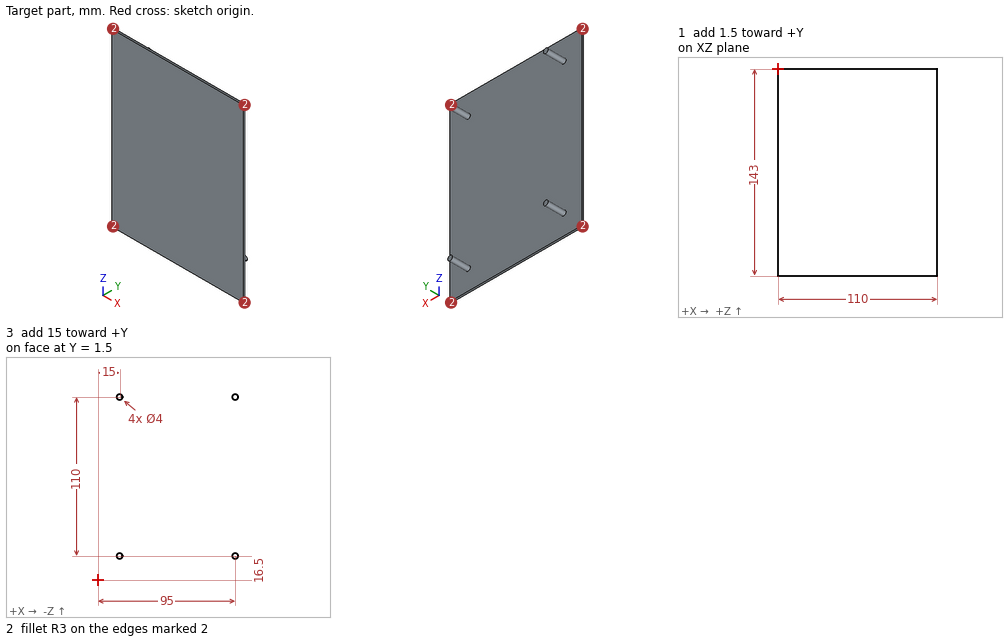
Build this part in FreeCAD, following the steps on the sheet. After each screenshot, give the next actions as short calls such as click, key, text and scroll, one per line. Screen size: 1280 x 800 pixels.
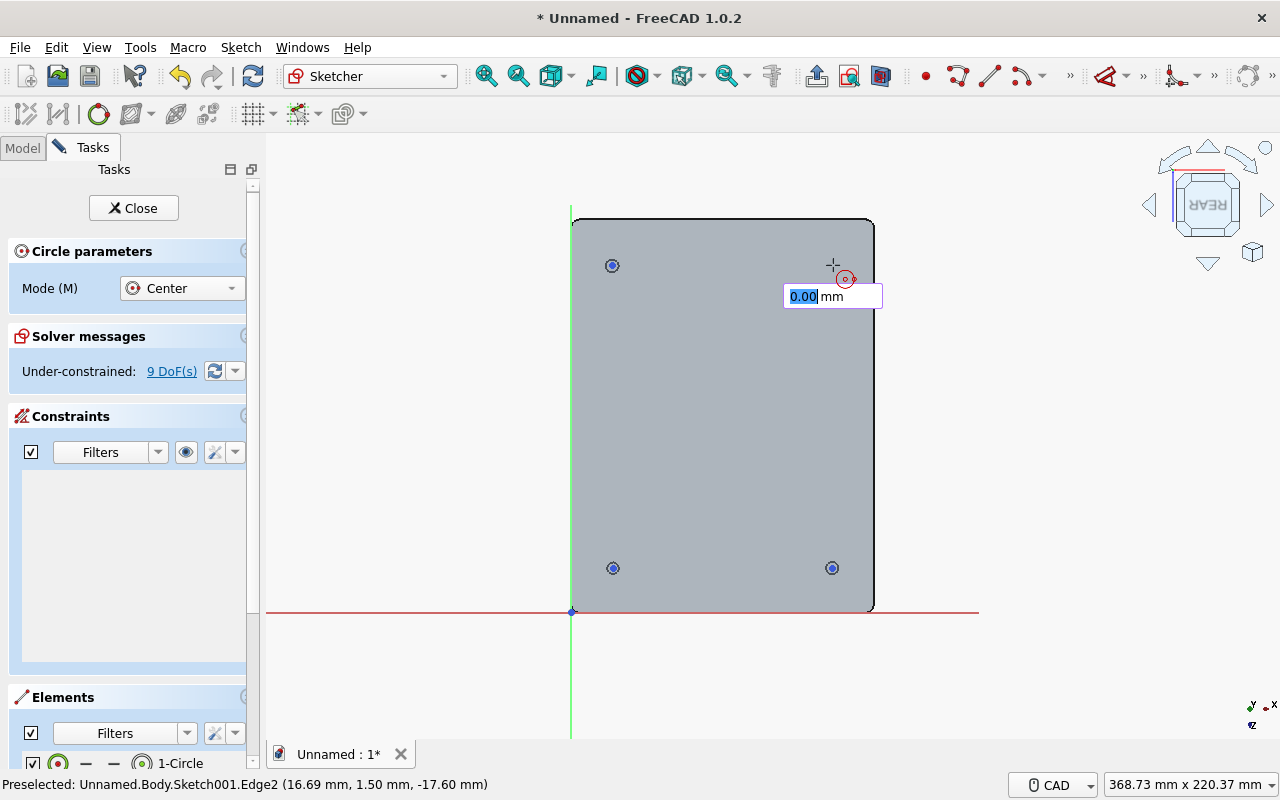
scroll(836, 261, up, 6)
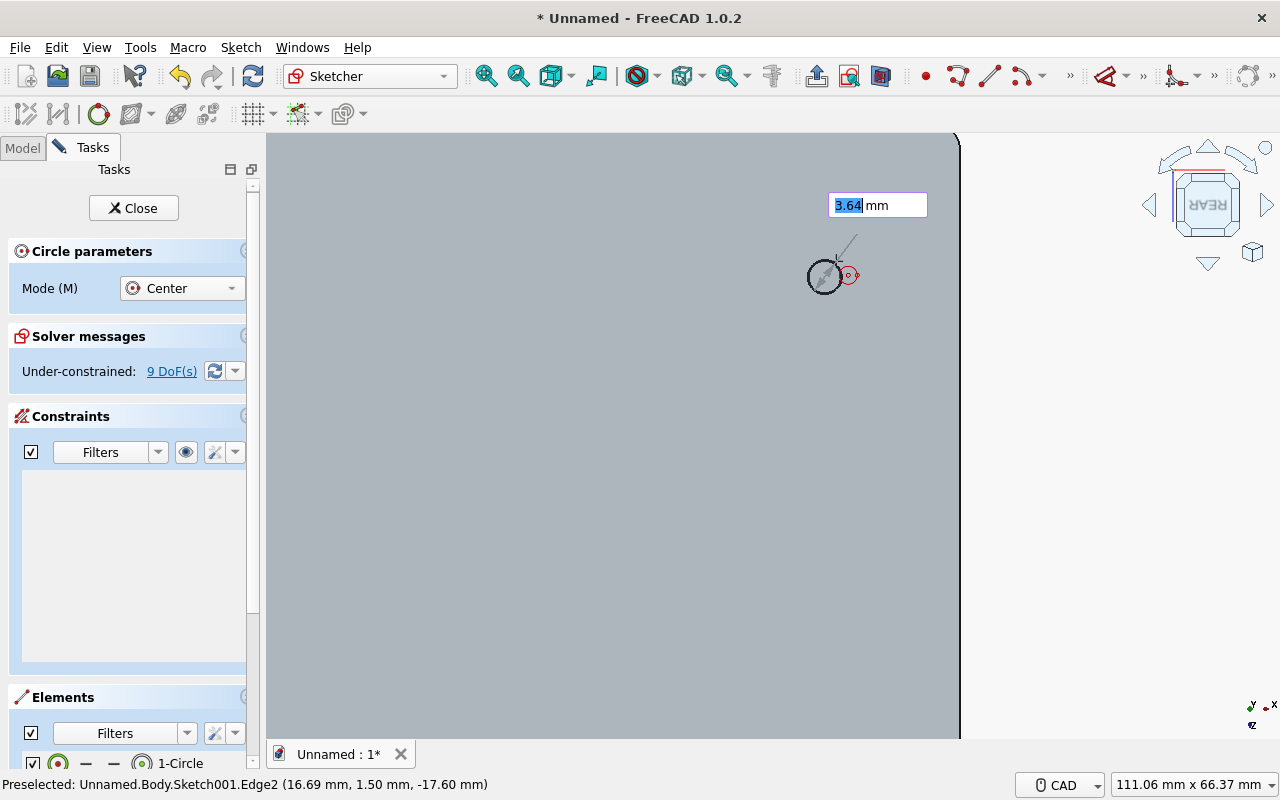
click(836, 260)
key(Escape)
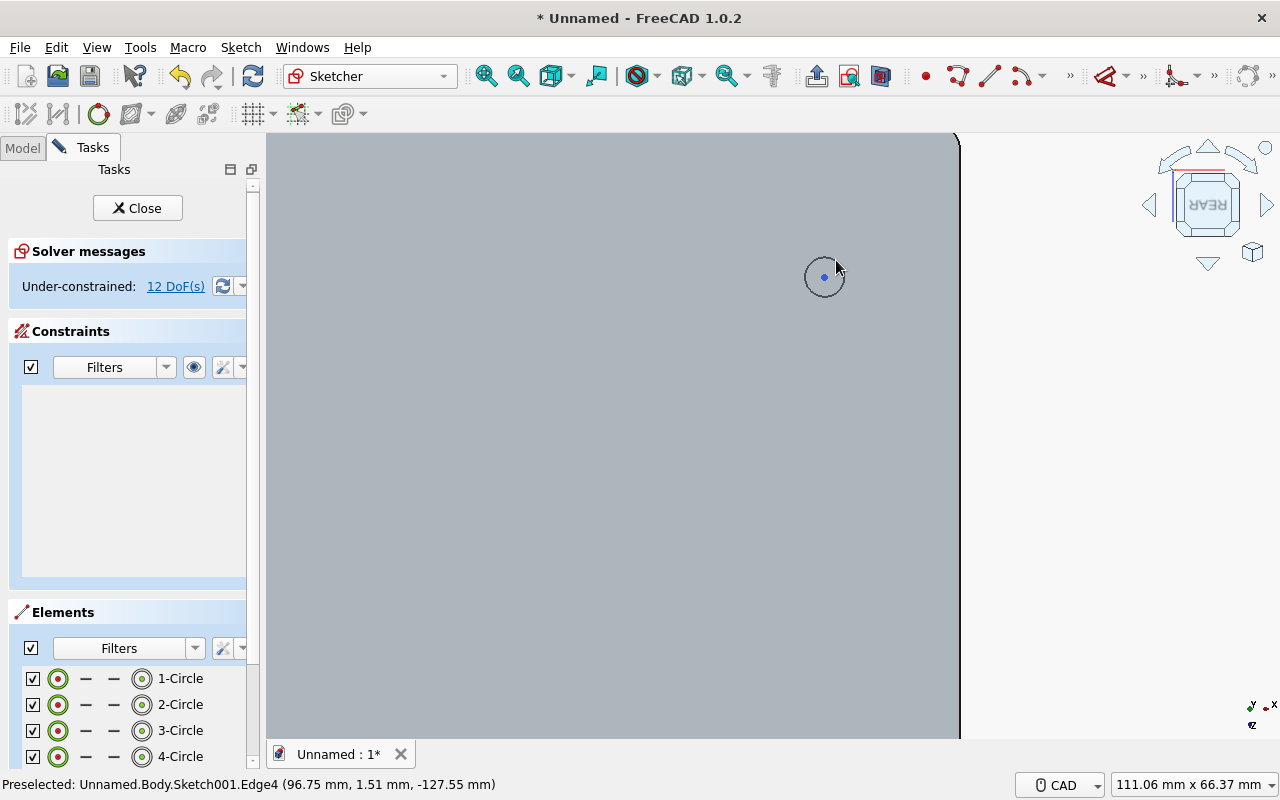
scroll(836, 261, down, 6)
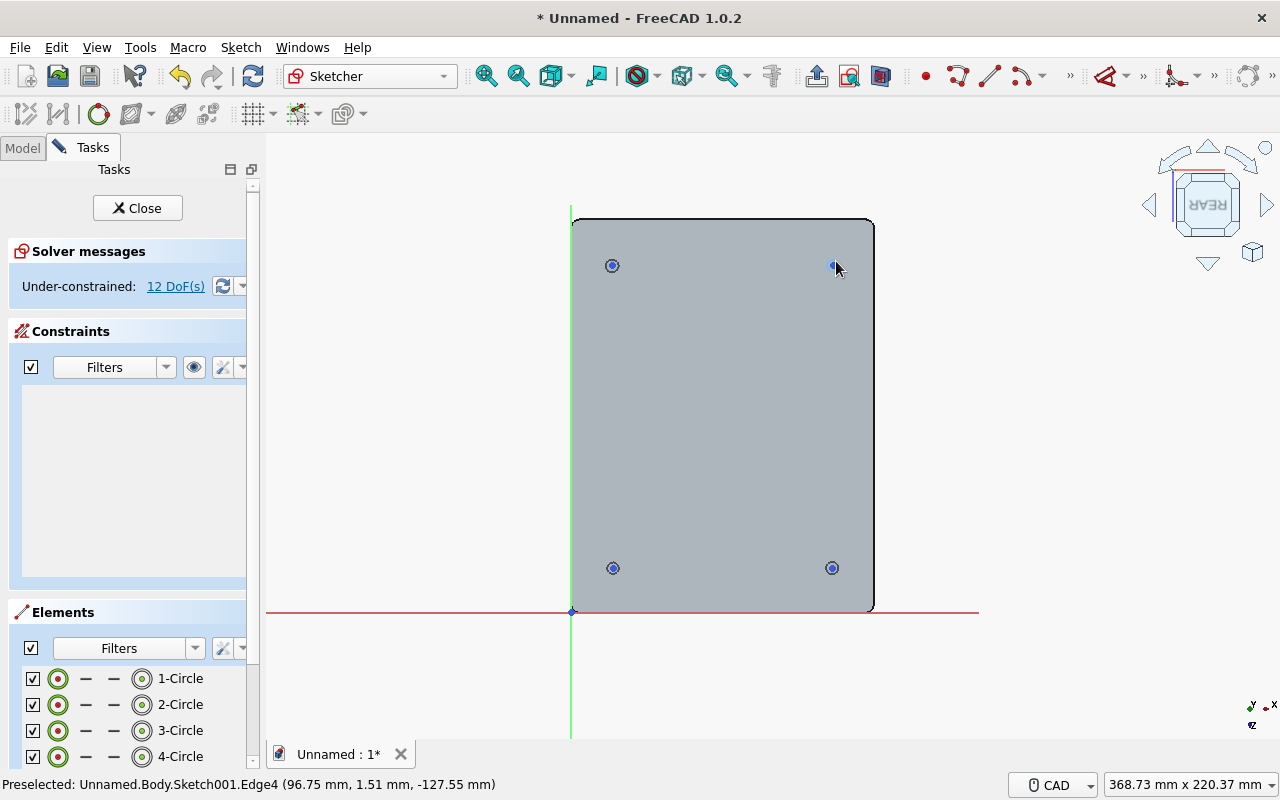
scroll(617, 261, up, 4)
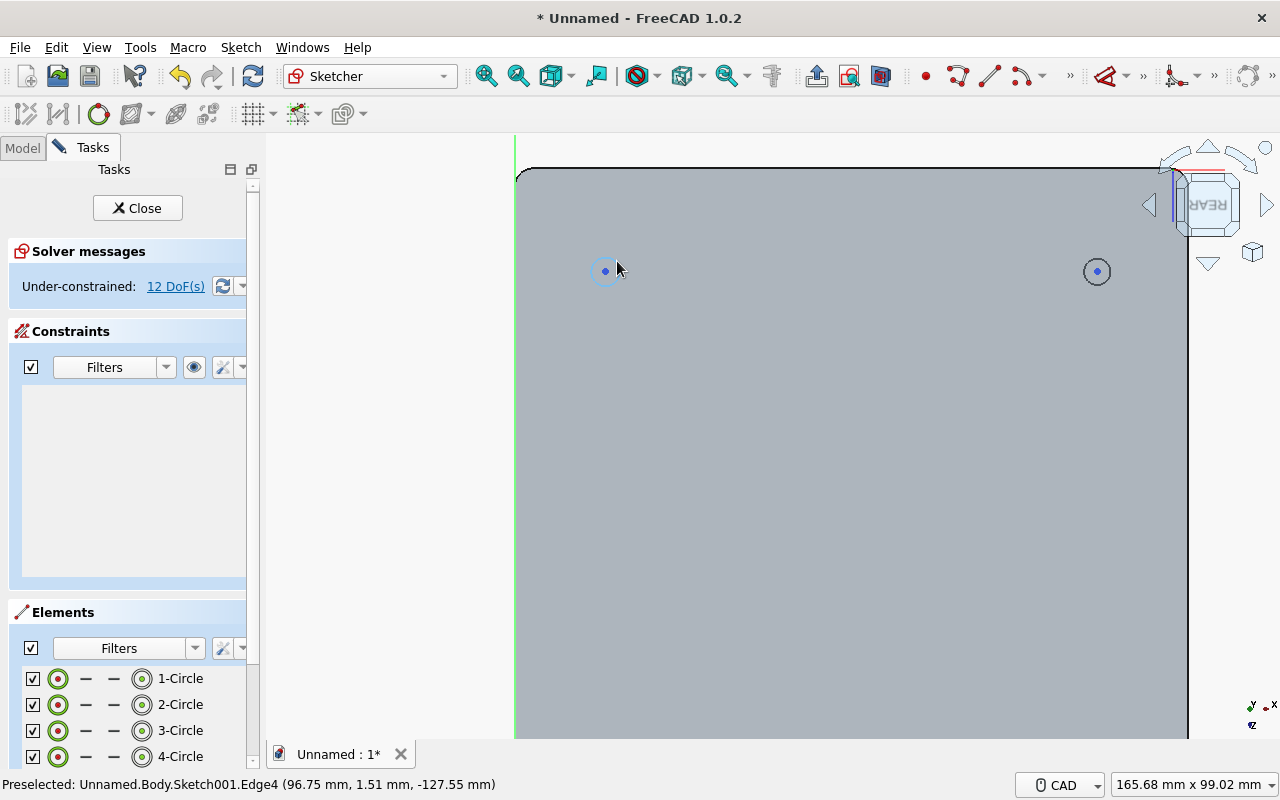
click(616, 262)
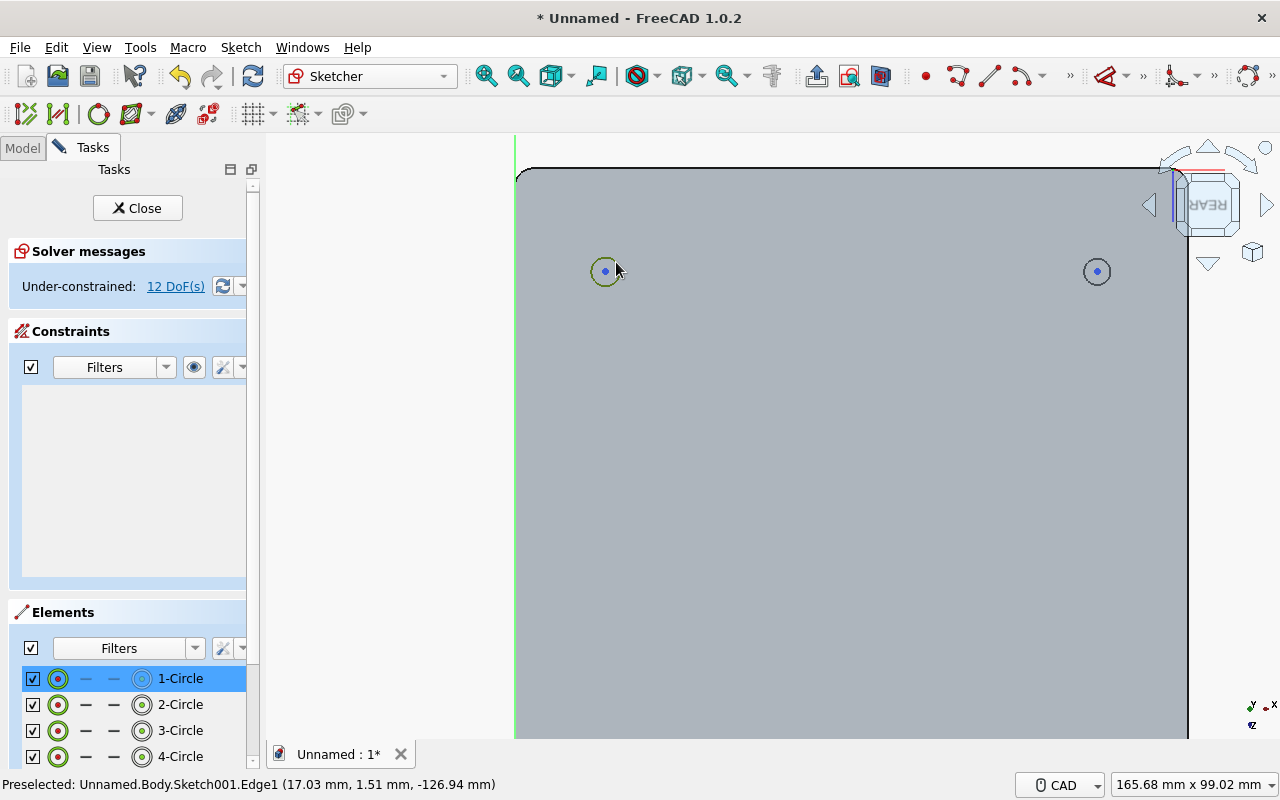
scroll(617, 261, down, 4)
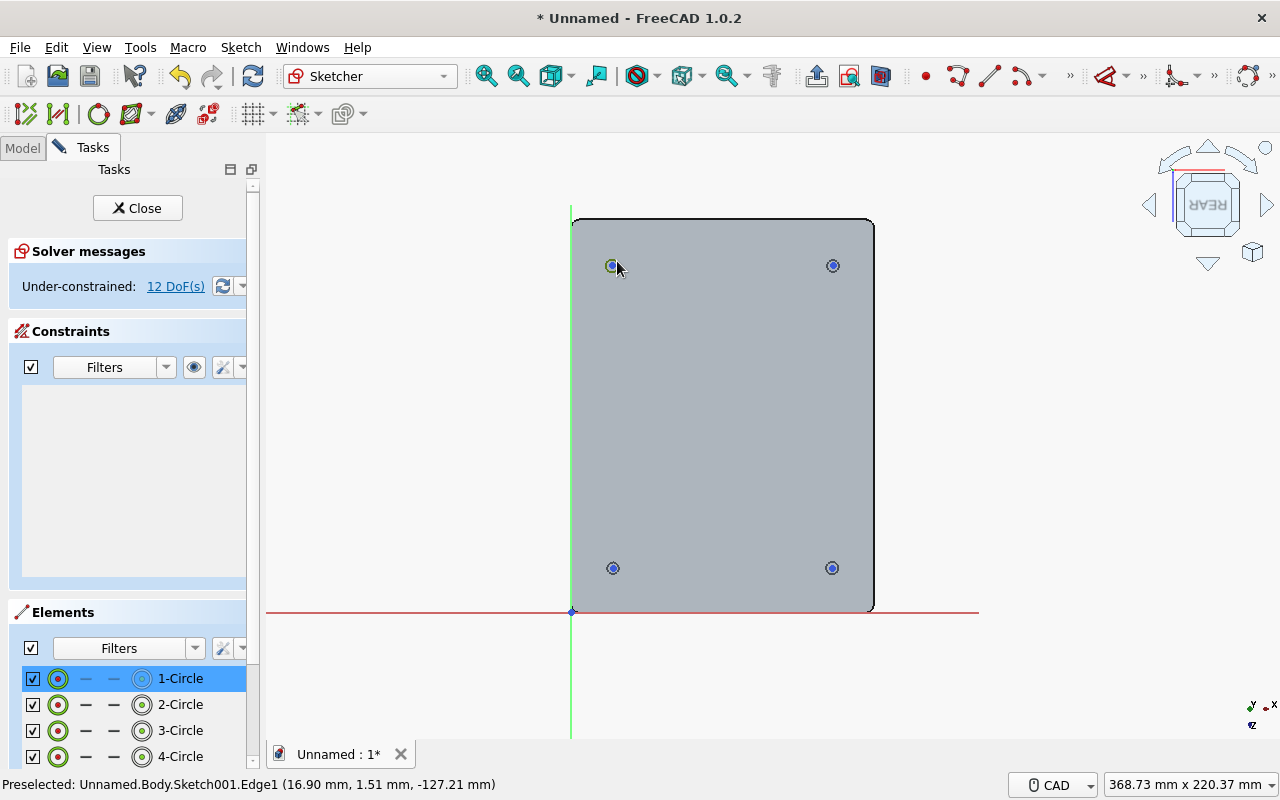
scroll(837, 564, up, 5)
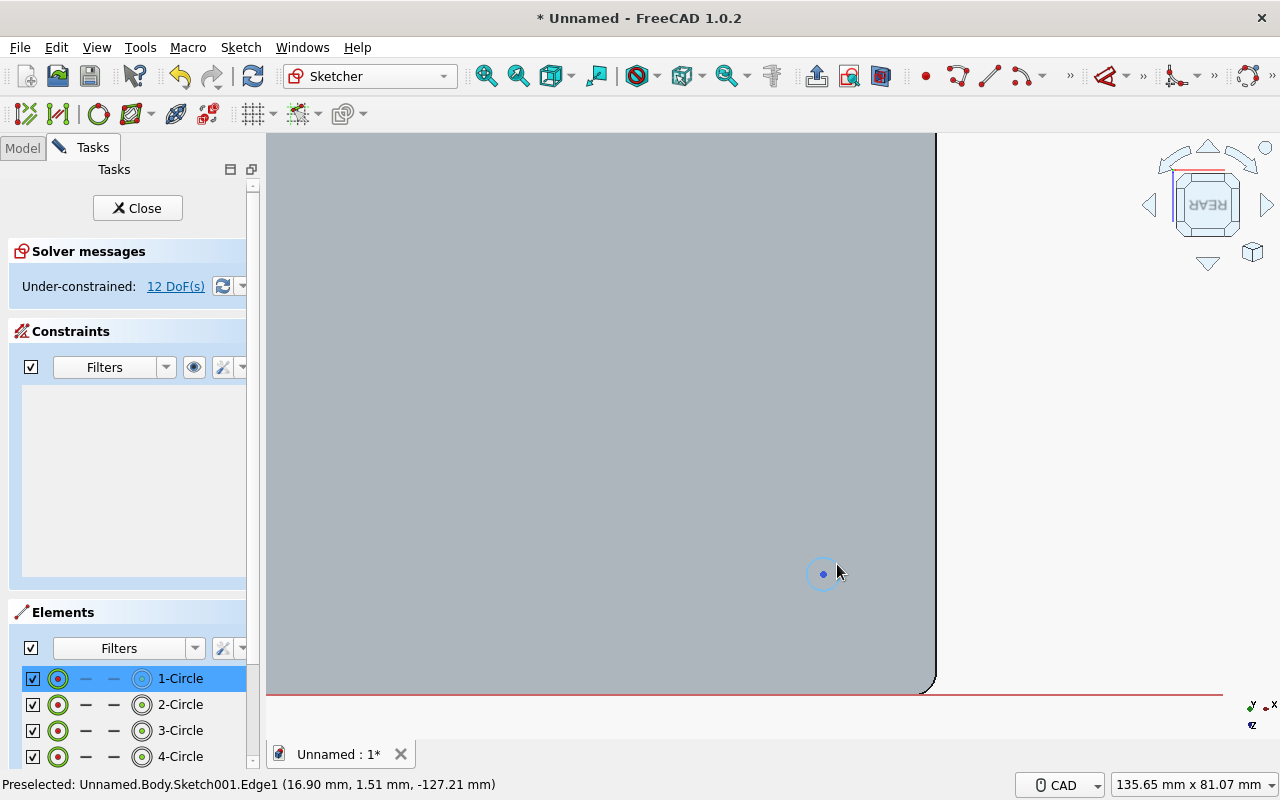
click(835, 562)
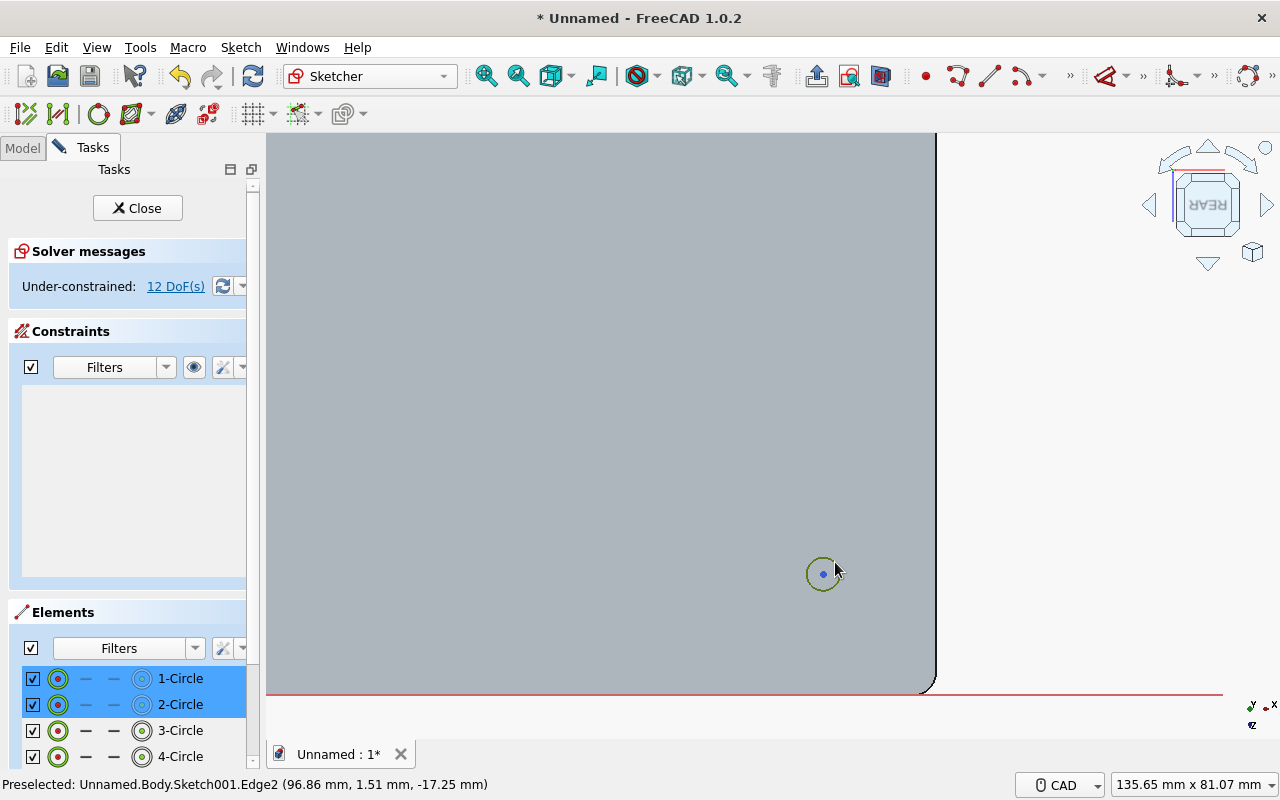
scroll(837, 565, down, 5)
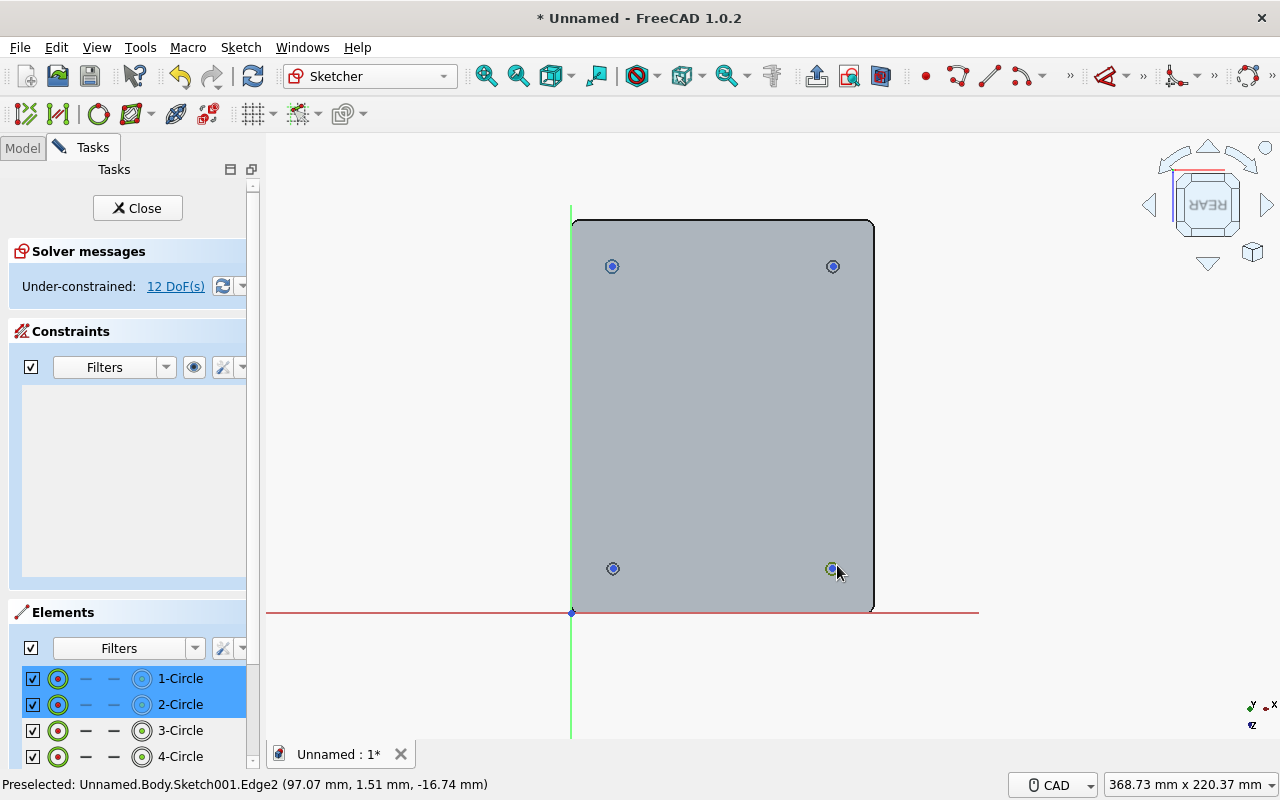
scroll(617, 565, up, 5)